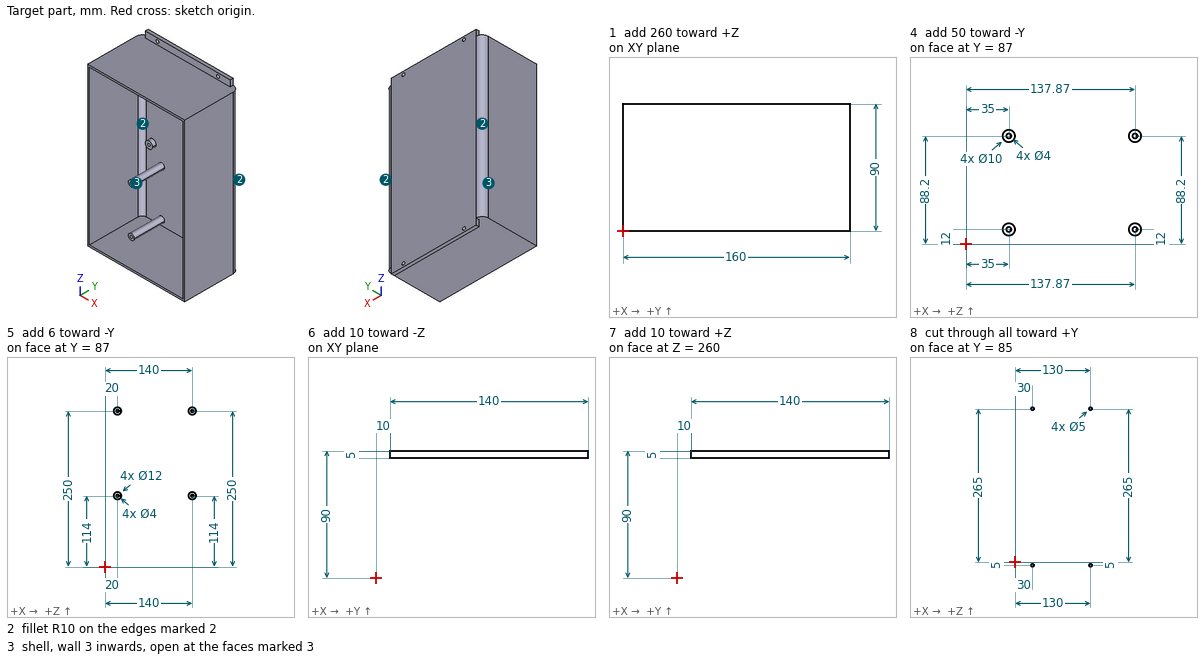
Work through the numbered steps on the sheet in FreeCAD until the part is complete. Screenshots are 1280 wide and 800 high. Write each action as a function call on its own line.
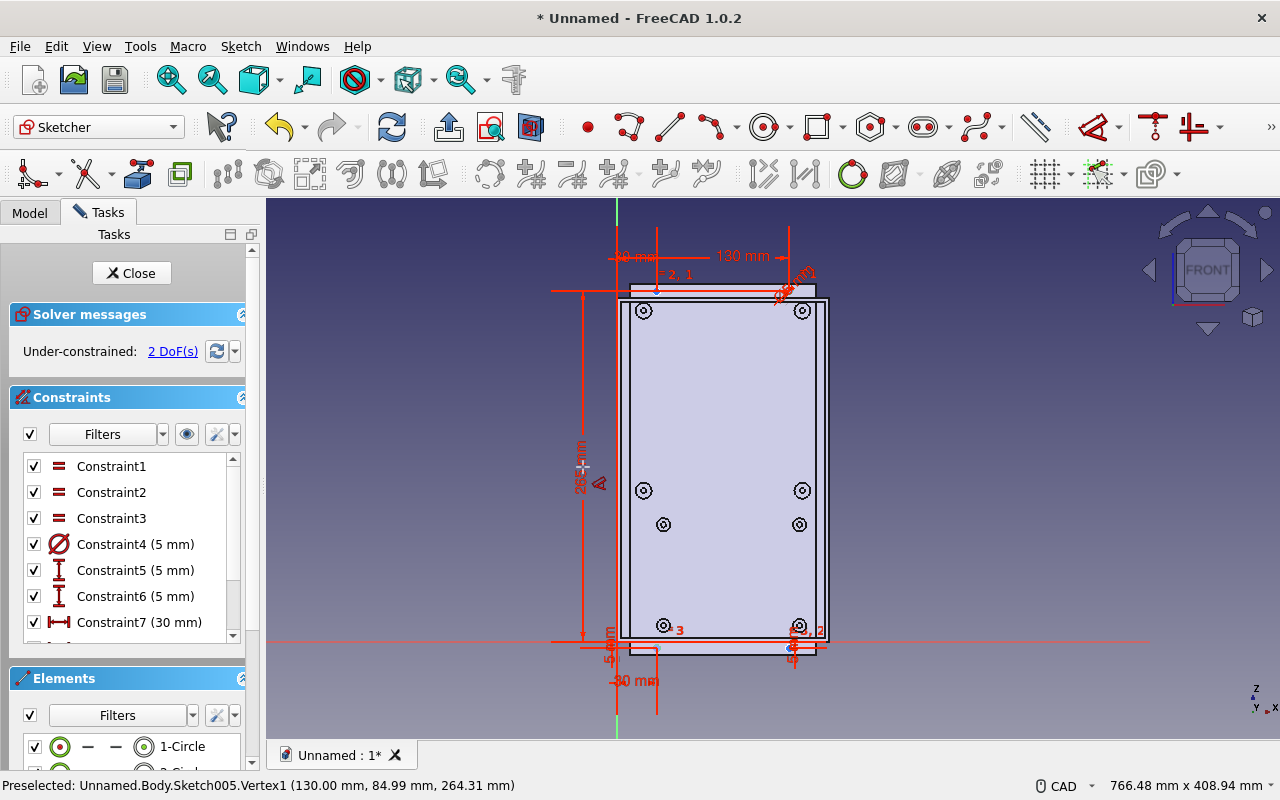
click(657, 292)
click(583, 386)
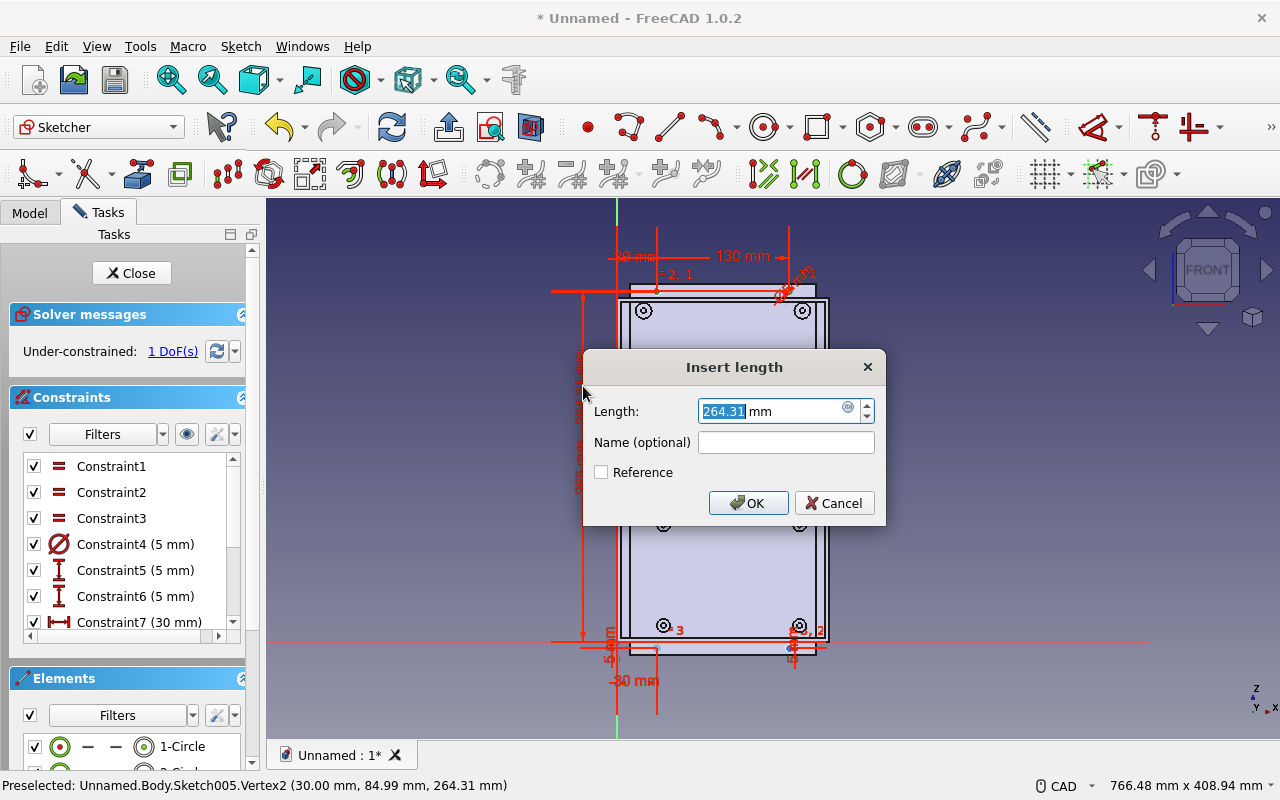
text(265)
key(Return)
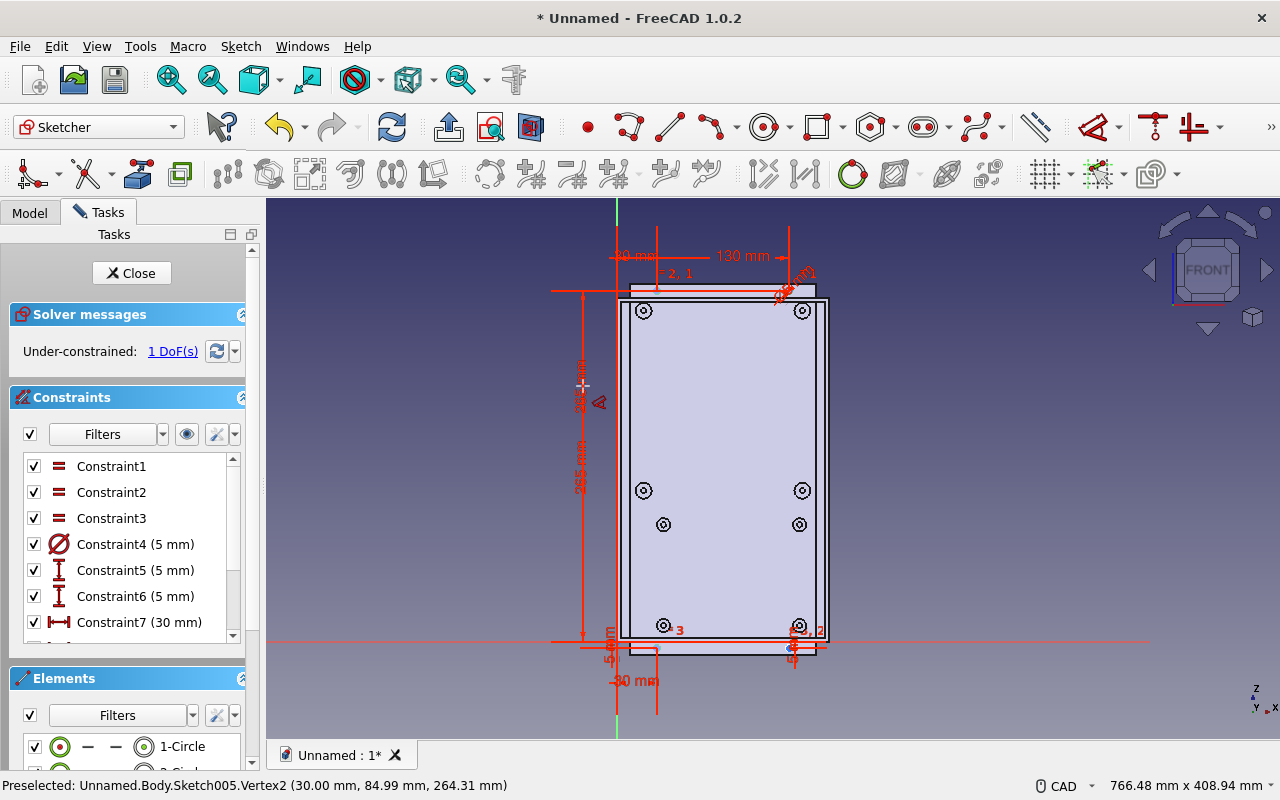
click(789, 648)
click(743, 682)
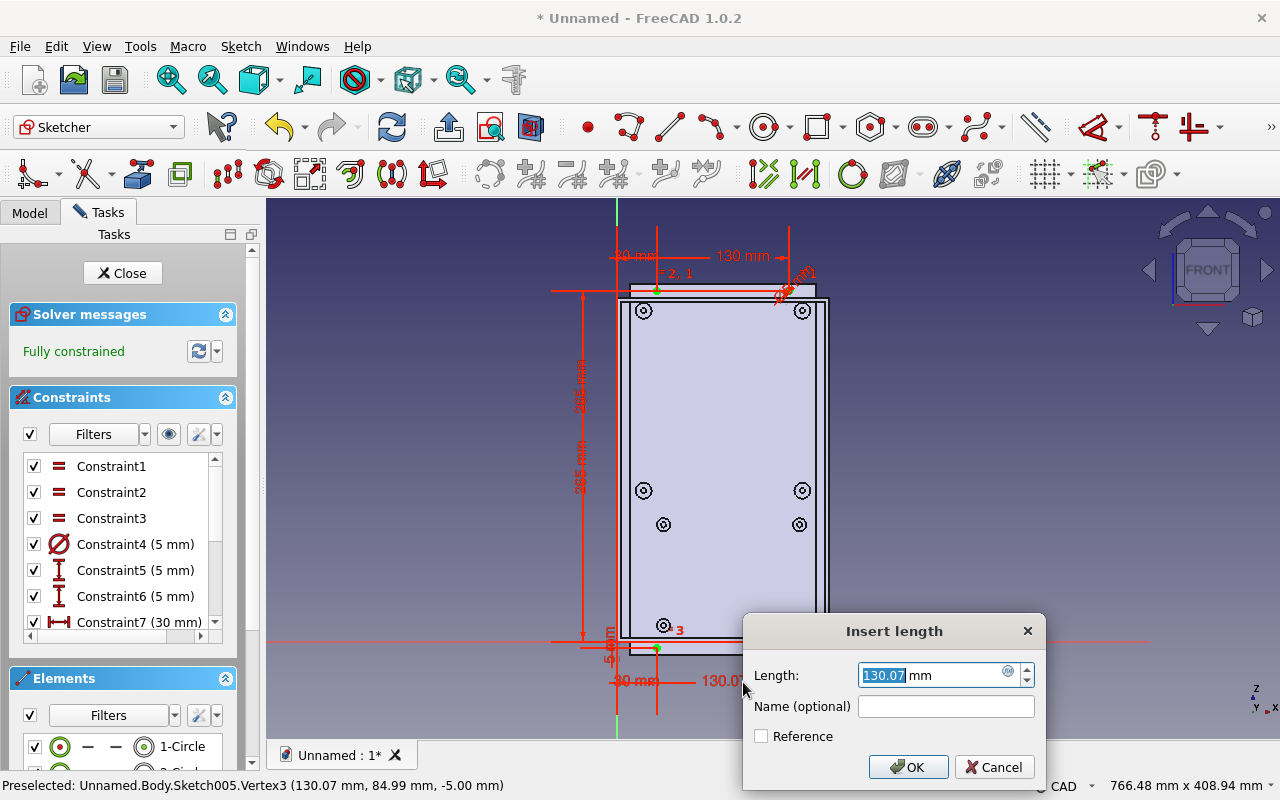
text(130)
key(Return)
key(Escape)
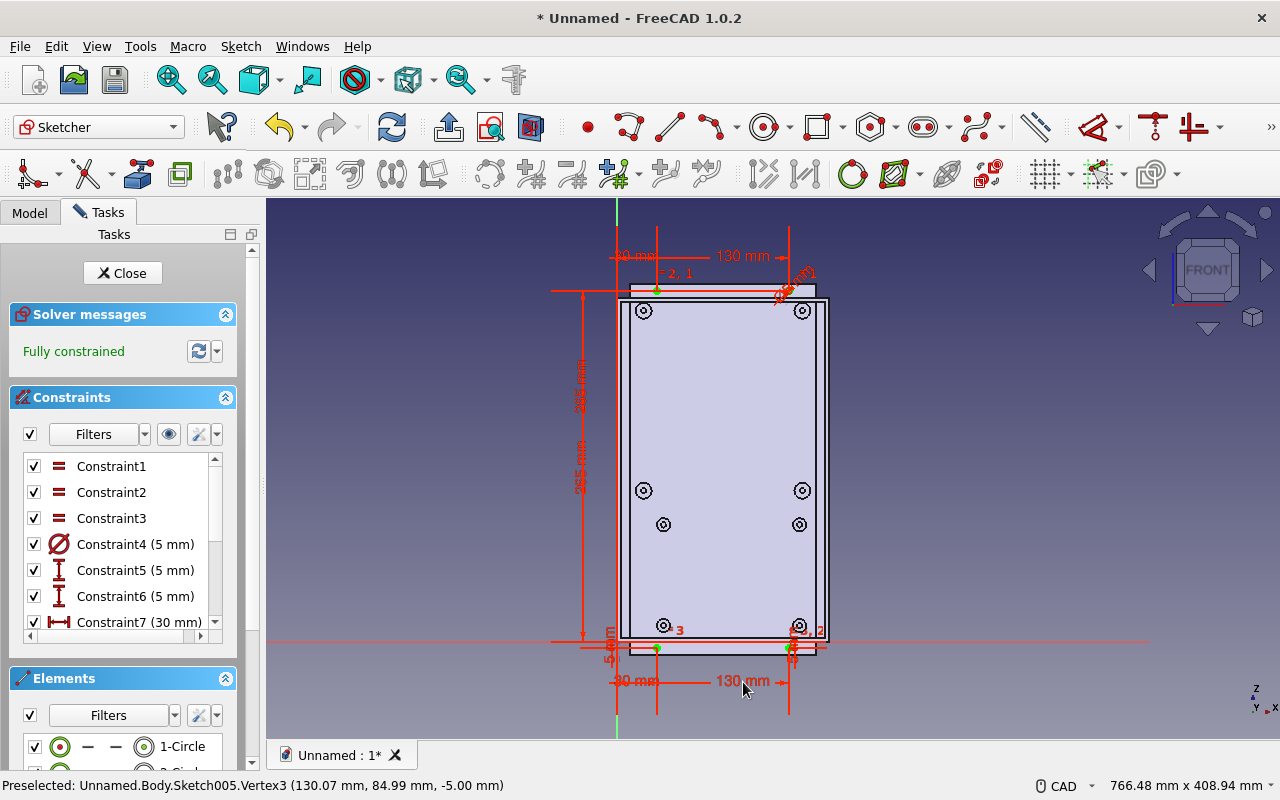
click(123, 273)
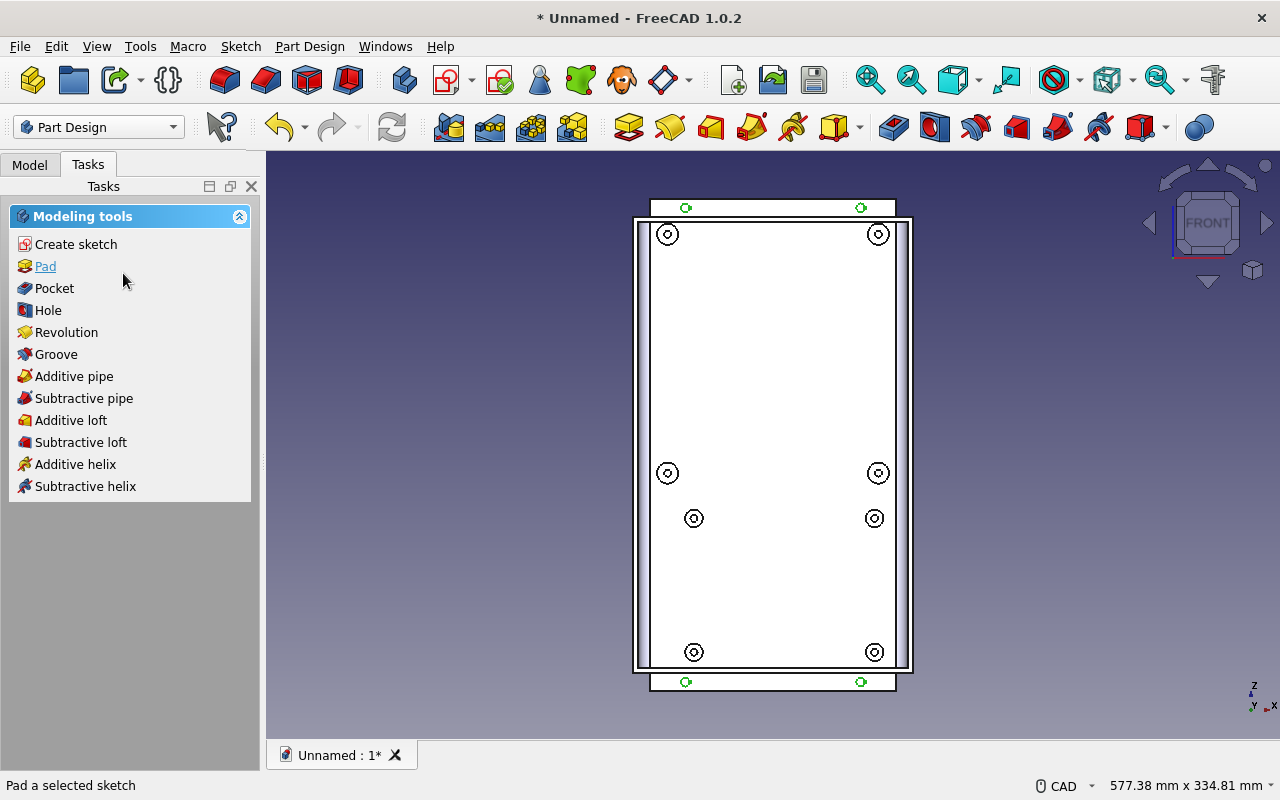
click(894, 128)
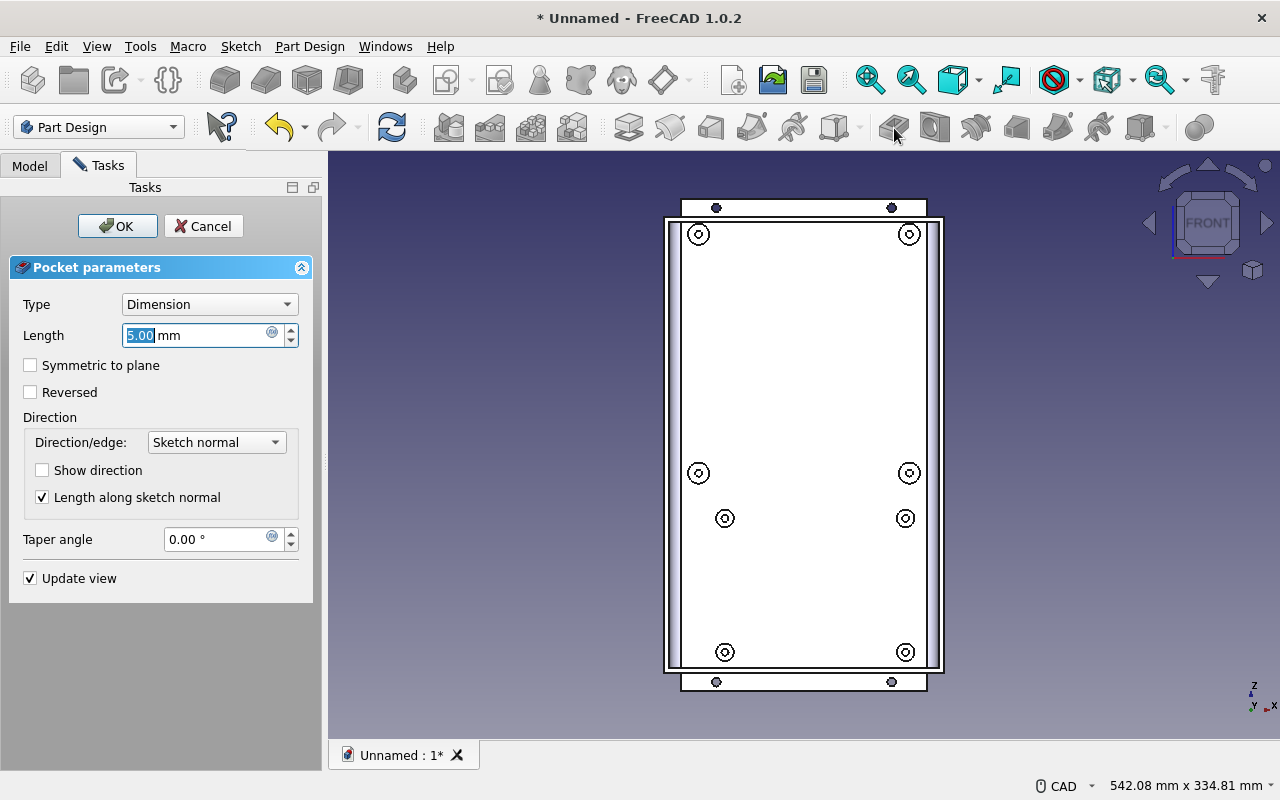
click(210, 304)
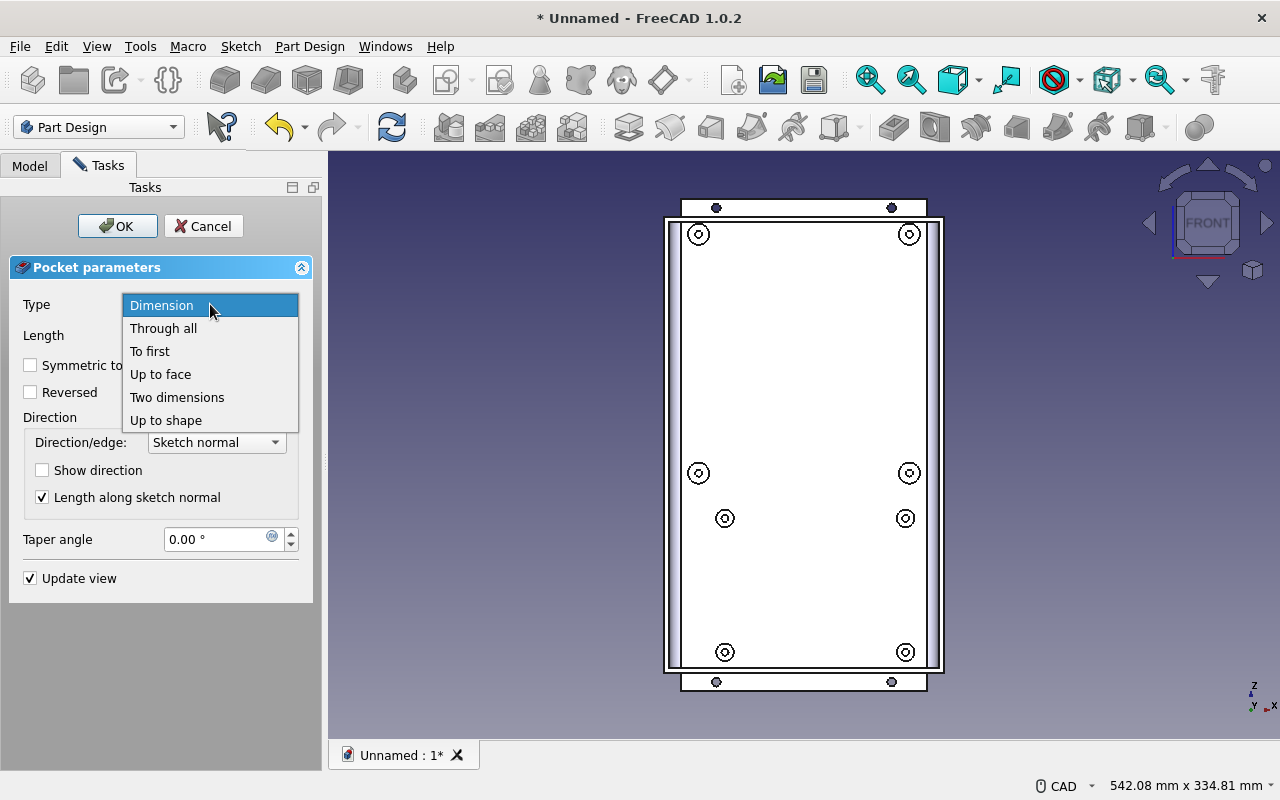
click(208, 328)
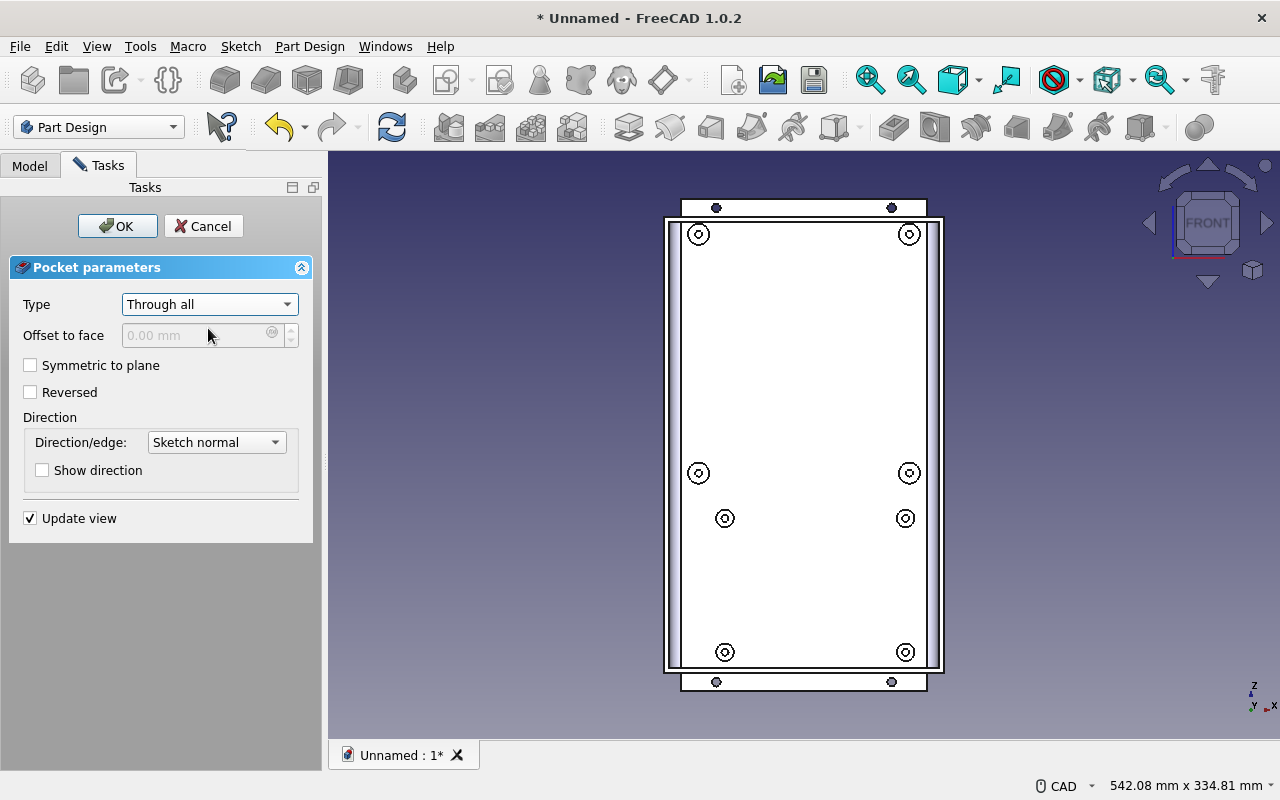
click(118, 226)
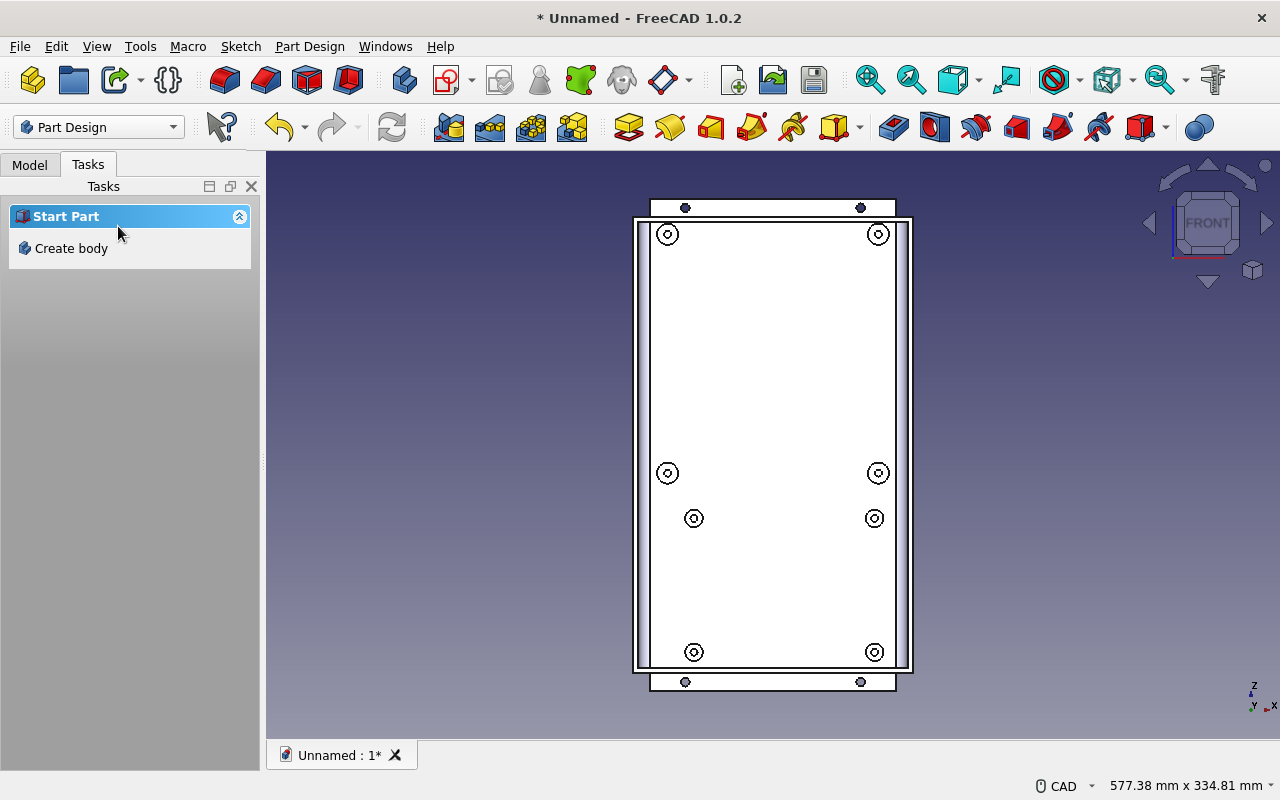
key(0)